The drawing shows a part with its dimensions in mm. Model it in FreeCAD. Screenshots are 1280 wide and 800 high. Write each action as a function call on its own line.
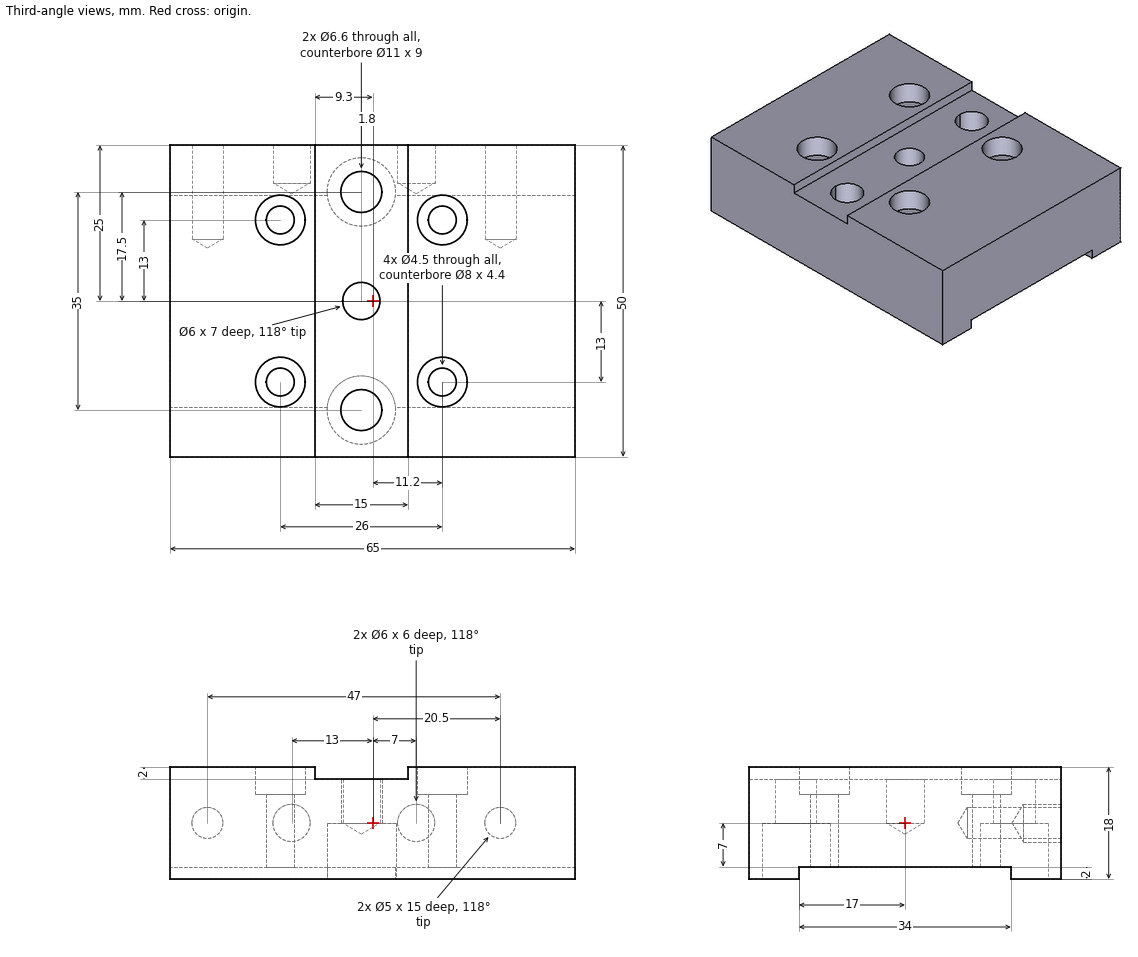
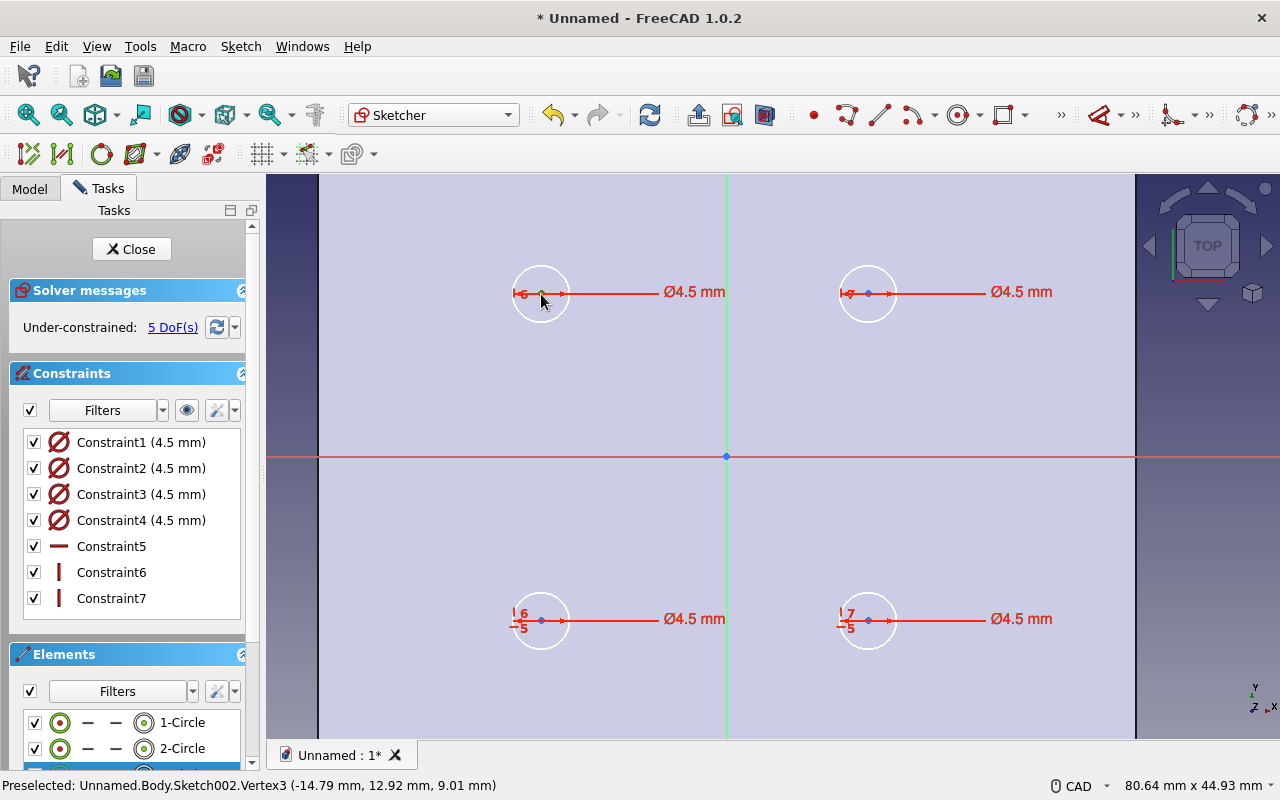
click(868, 294)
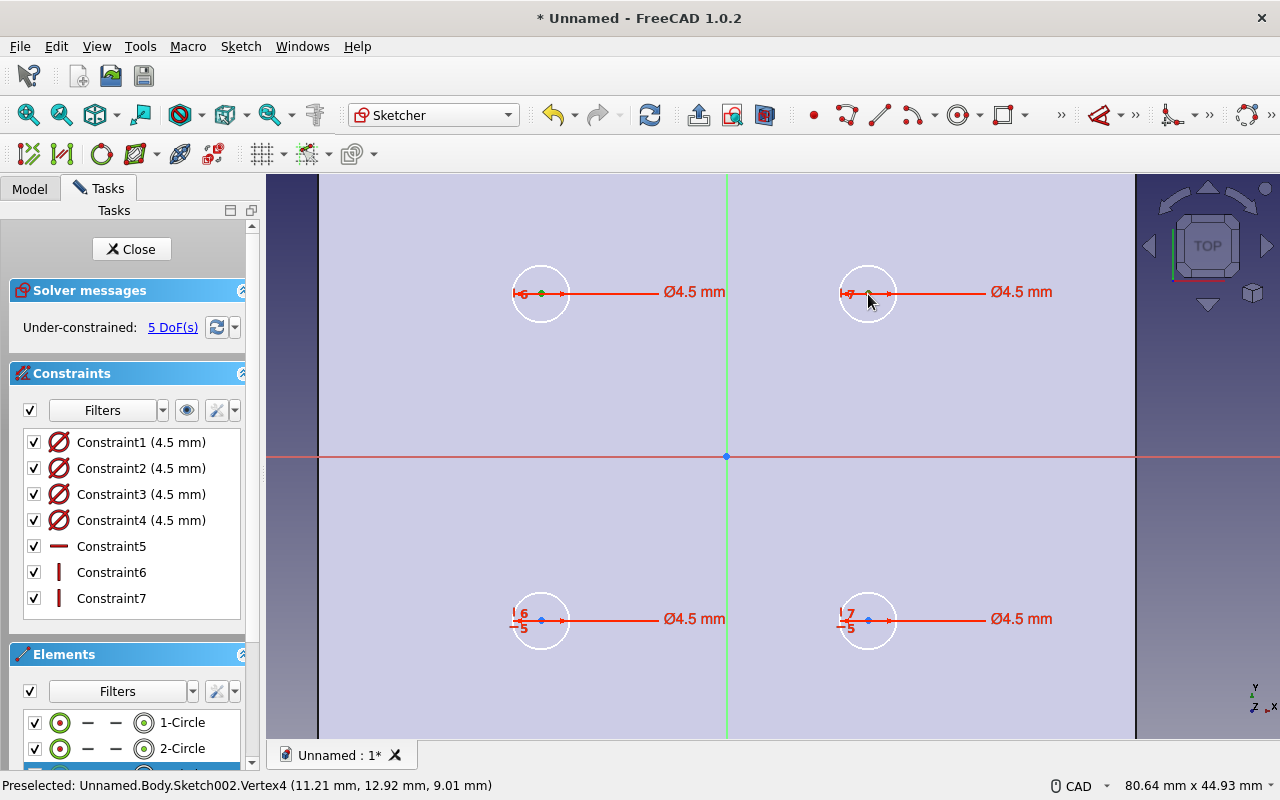
key(h)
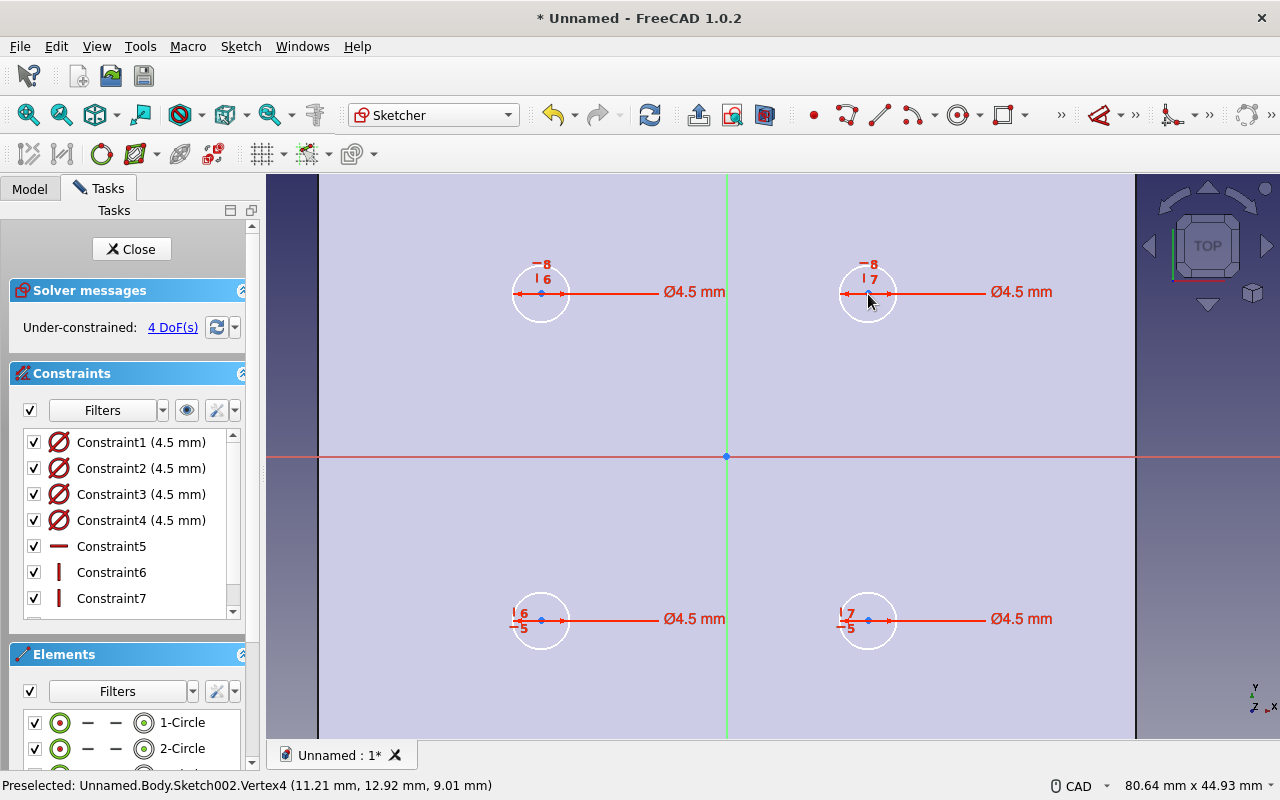
key(d)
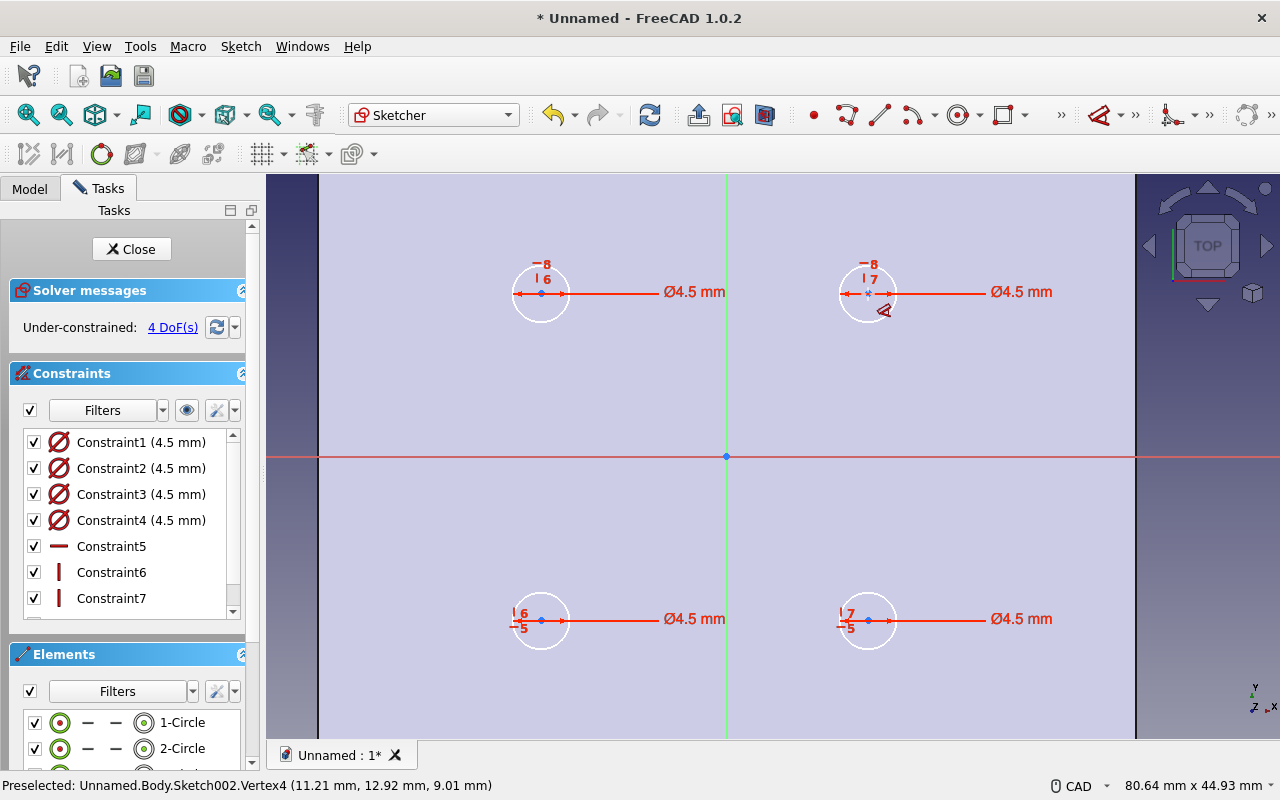
click(868, 621)
click(902, 539)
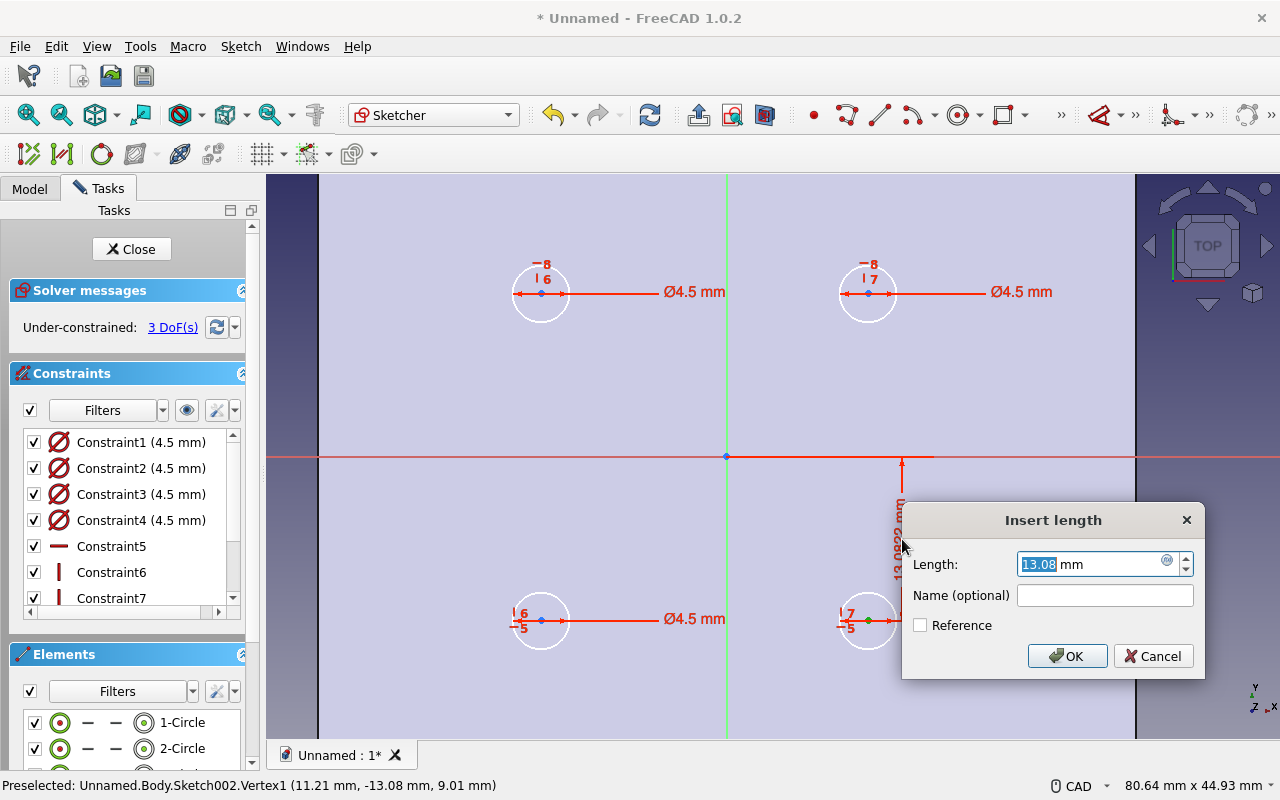
text(13)
key(Return)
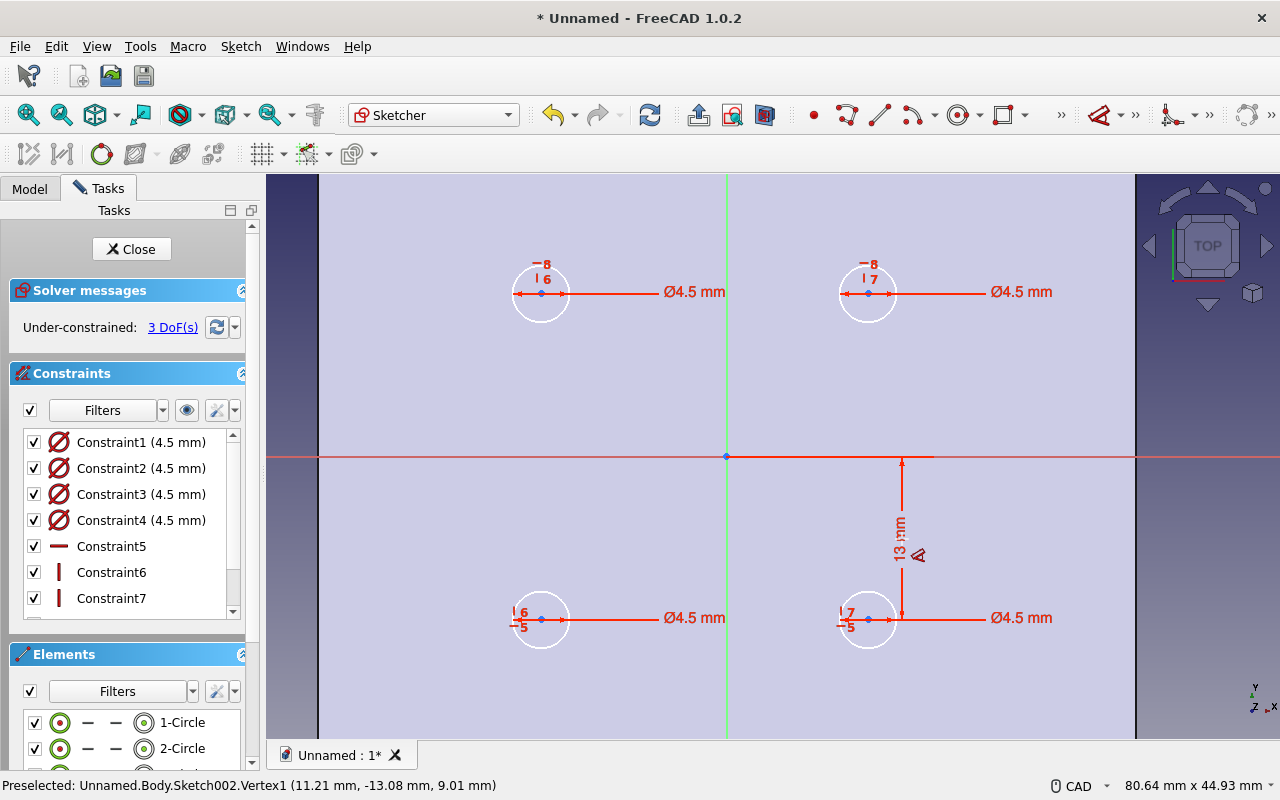
click(541, 294)
click(507, 375)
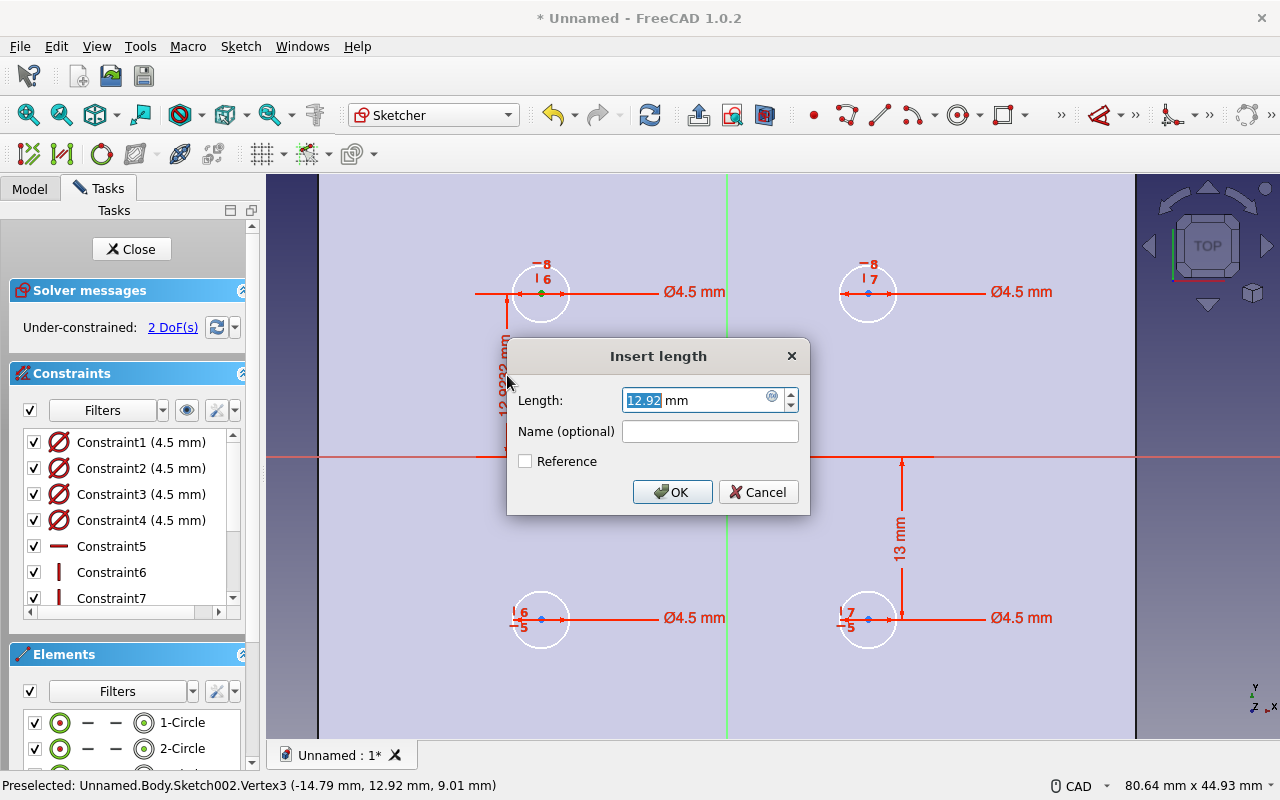
text(13)
key(Return)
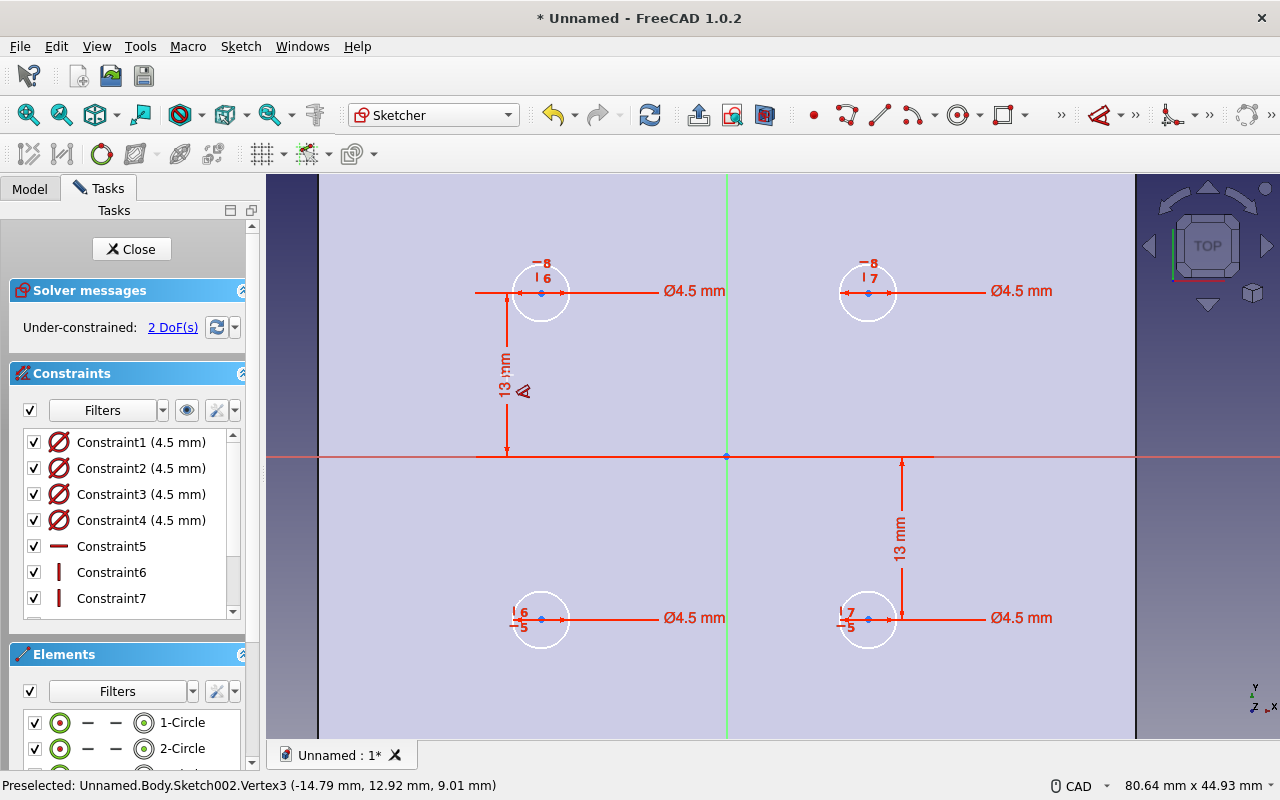
click(868, 620)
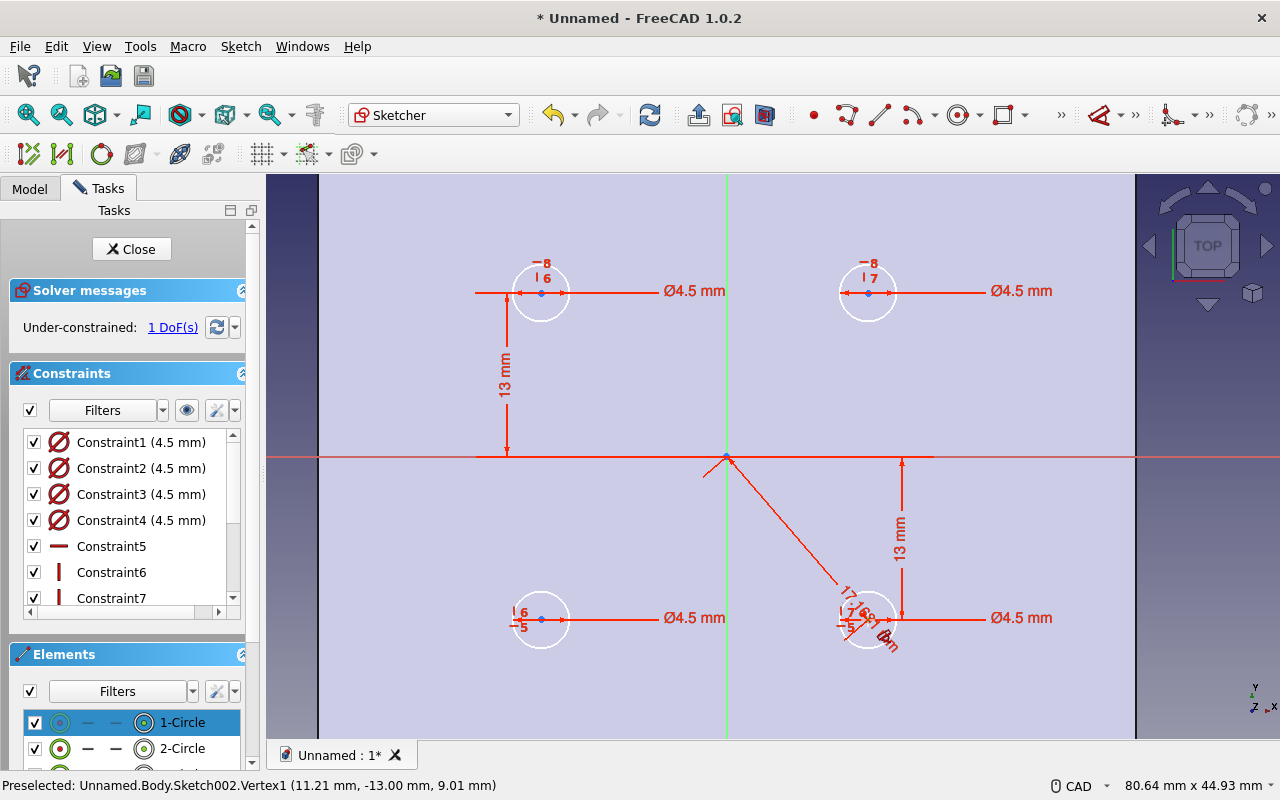
click(541, 620)
click(705, 654)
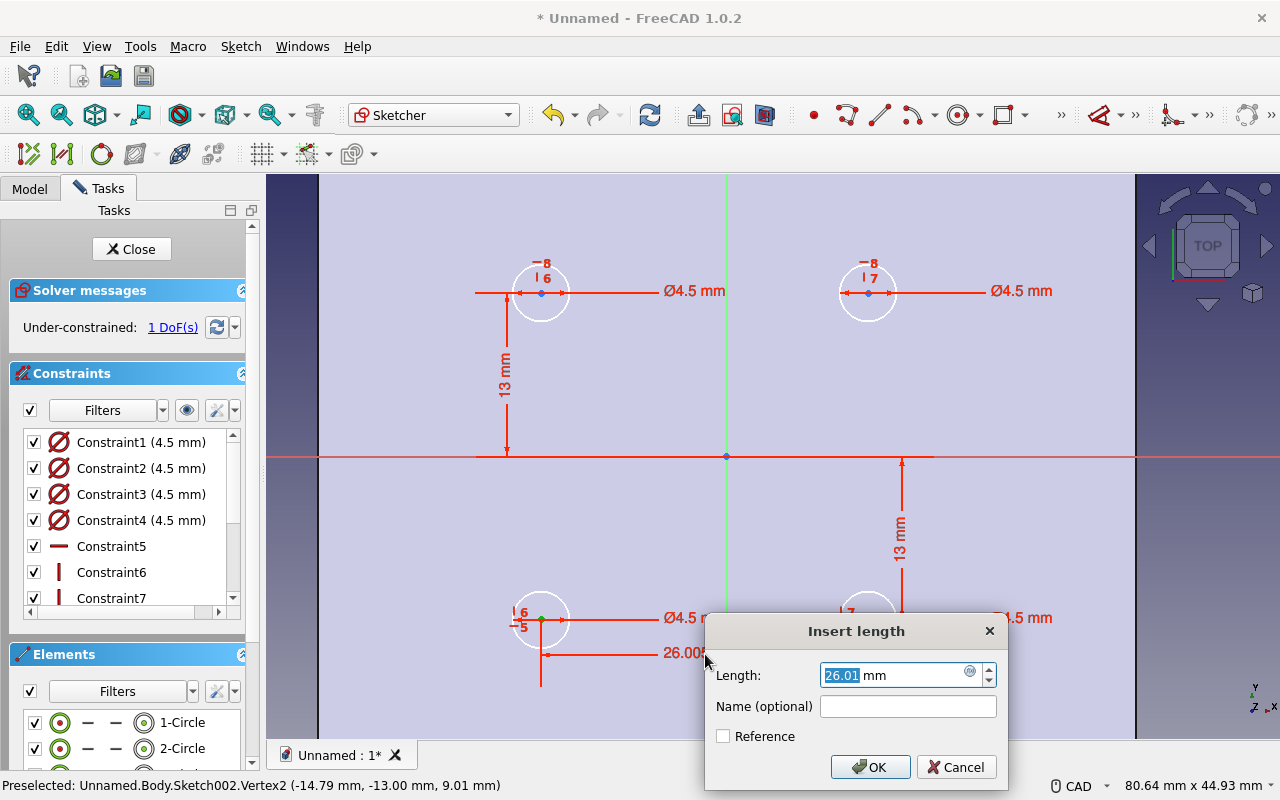
text(26)
key(Return)